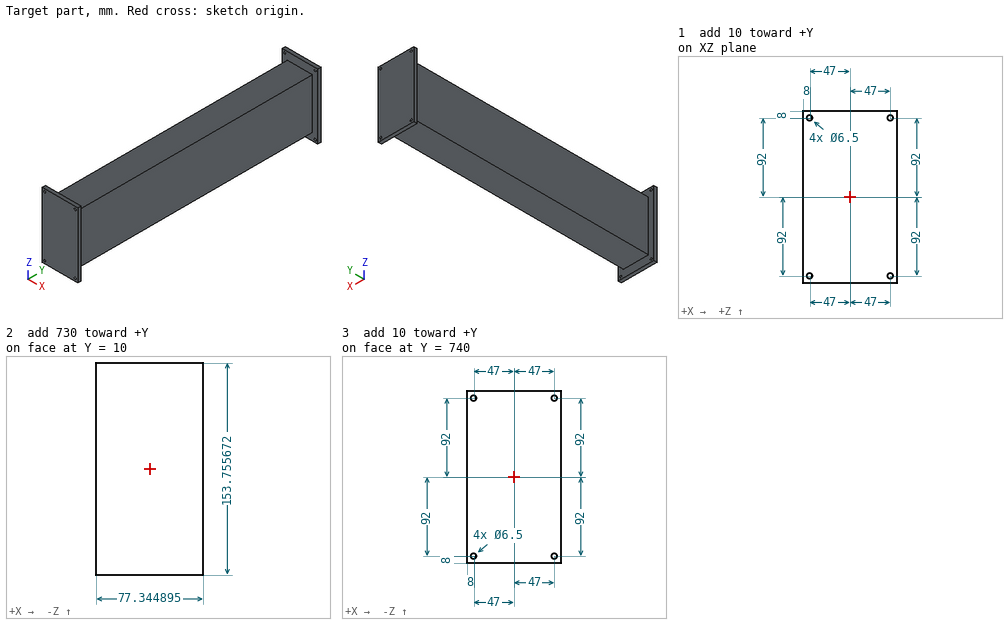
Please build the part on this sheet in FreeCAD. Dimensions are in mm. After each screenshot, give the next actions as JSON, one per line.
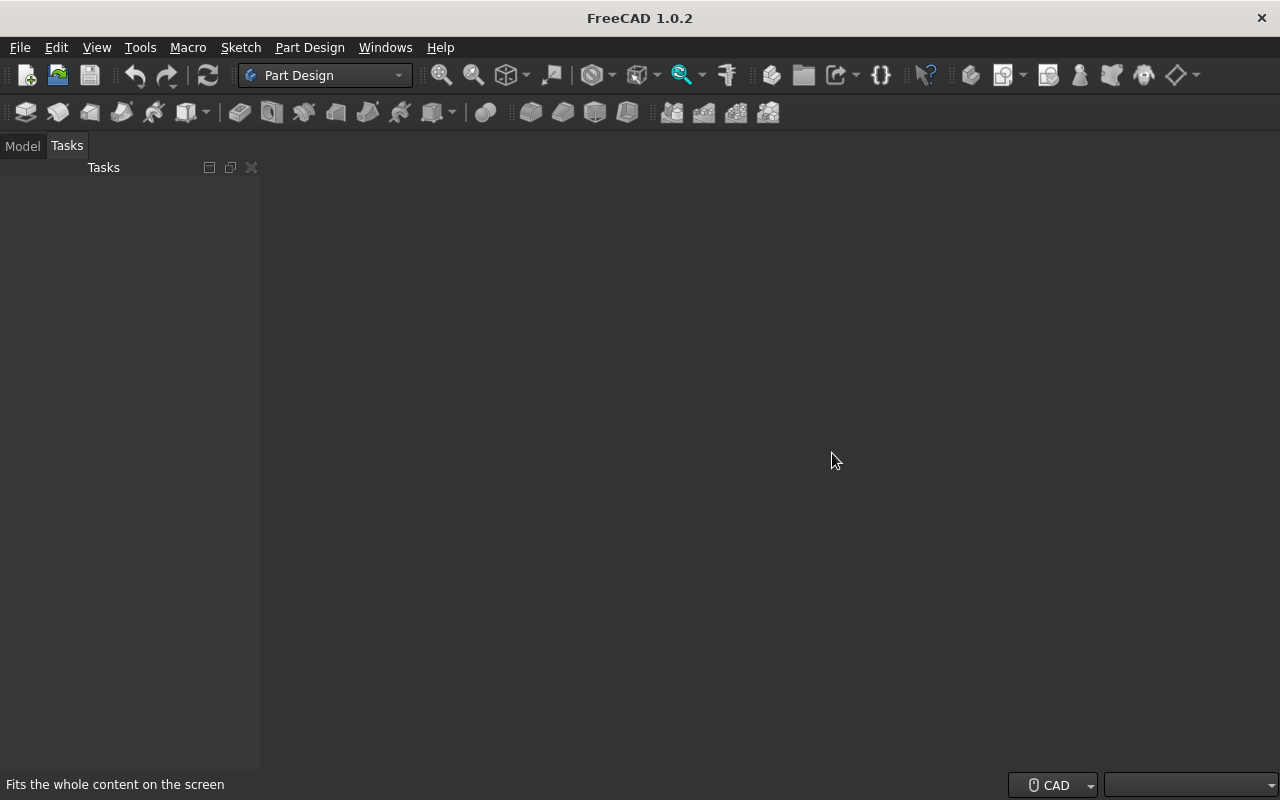
{"action": "left_click", "coordinate": [26, 76]}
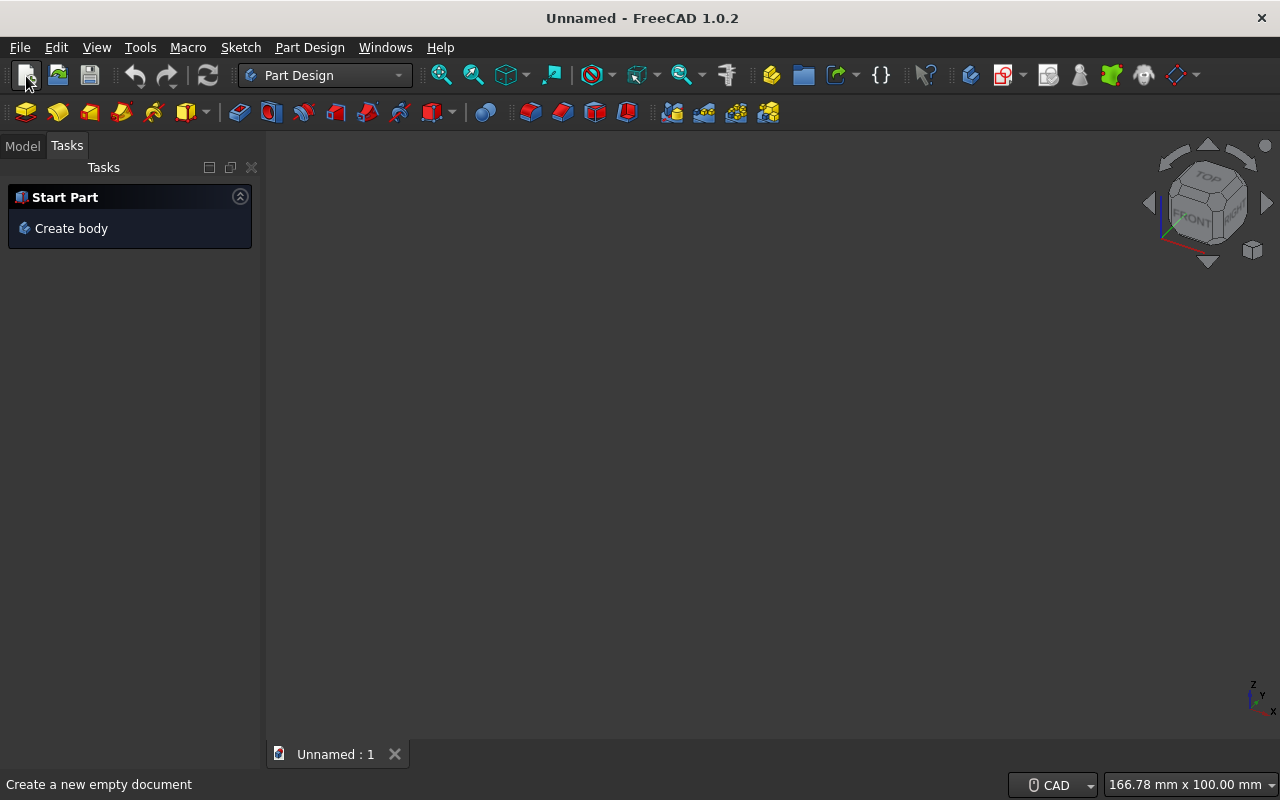
{"action": "left_click", "coordinate": [1004, 76]}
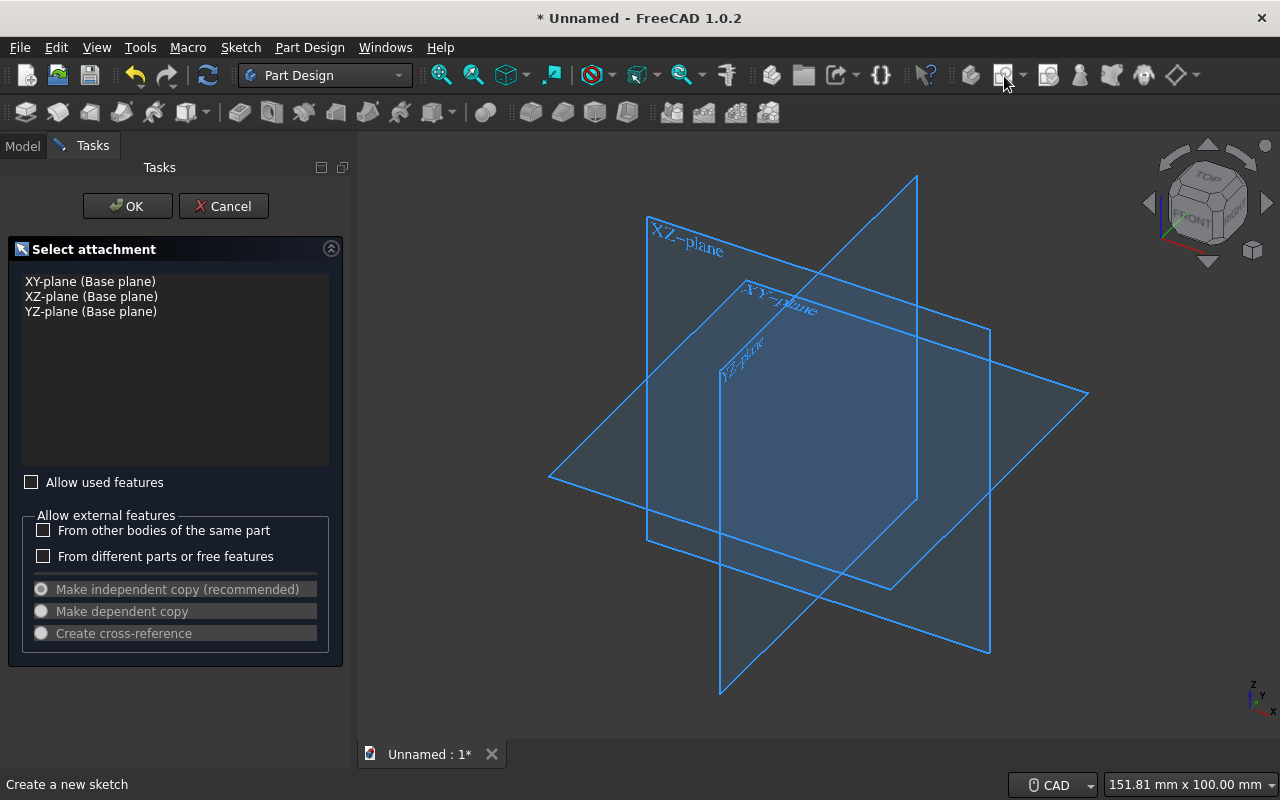
{"action": "left_click", "coordinate": [82, 296]}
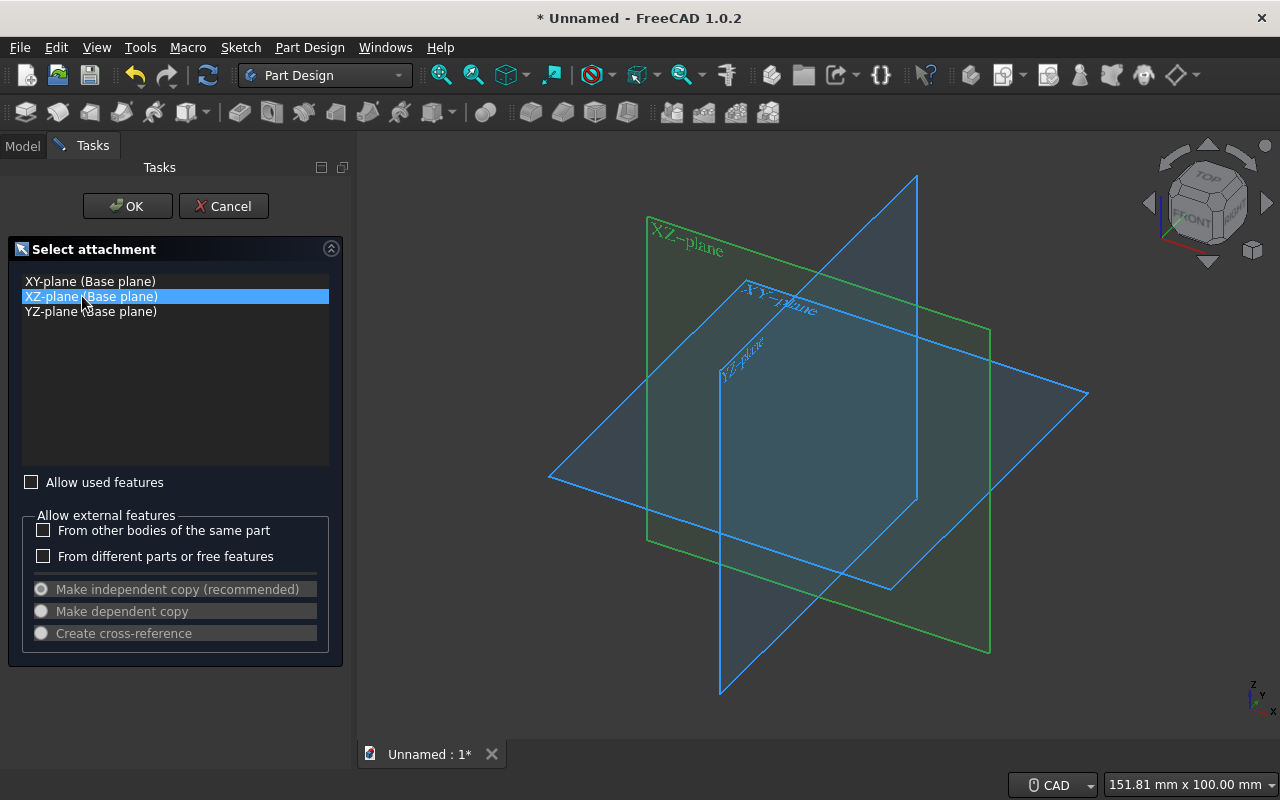
{"action": "left_click", "coordinate": [128, 206]}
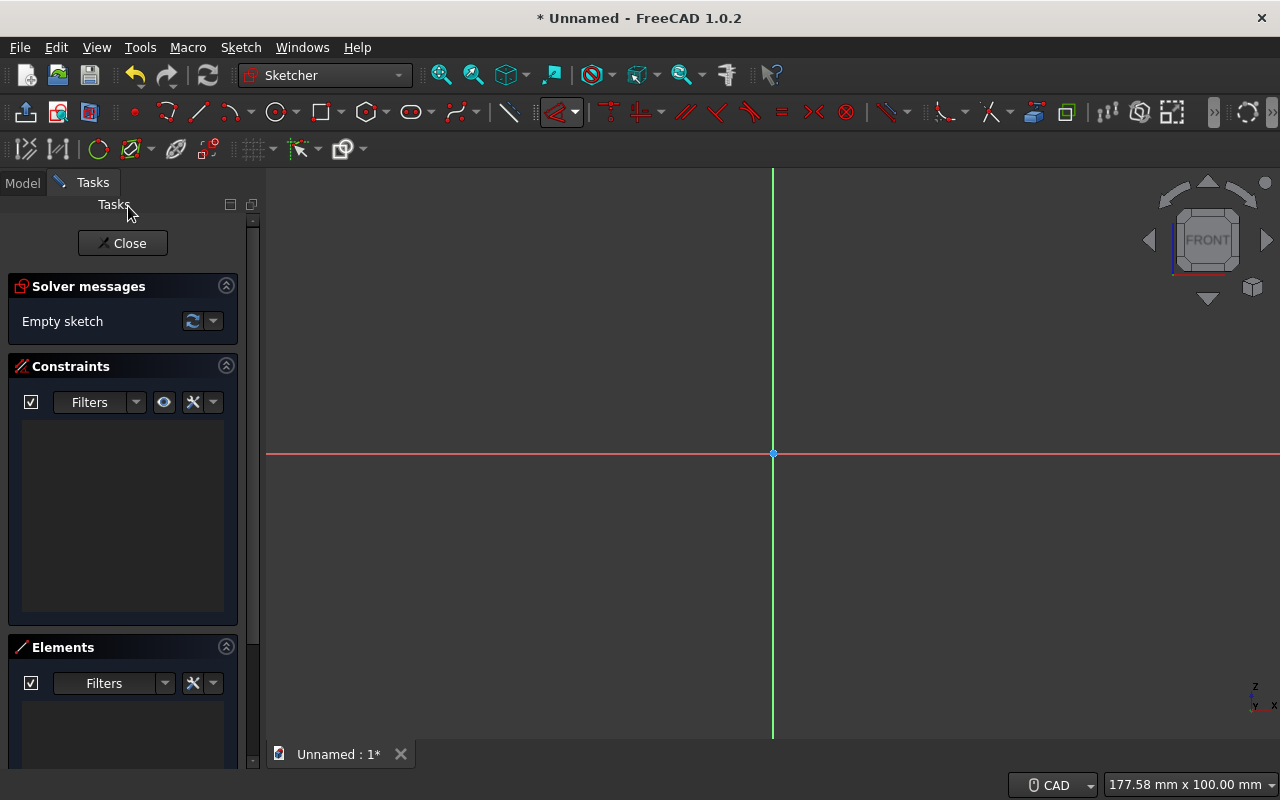
{"action": "scroll", "coordinate": [675, 453], "scroll_direction": "down", "scroll_amount": 6}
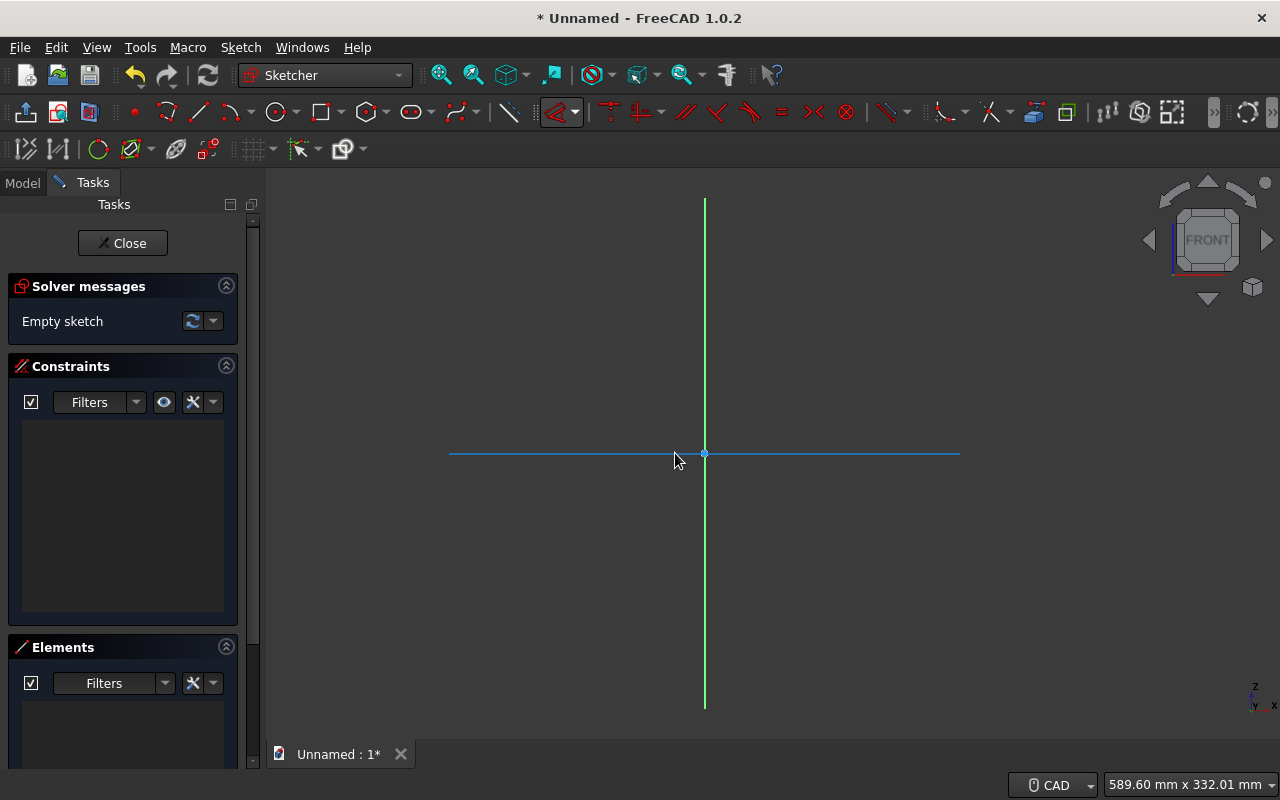
{"action": "left_click", "coordinate": [344, 112]}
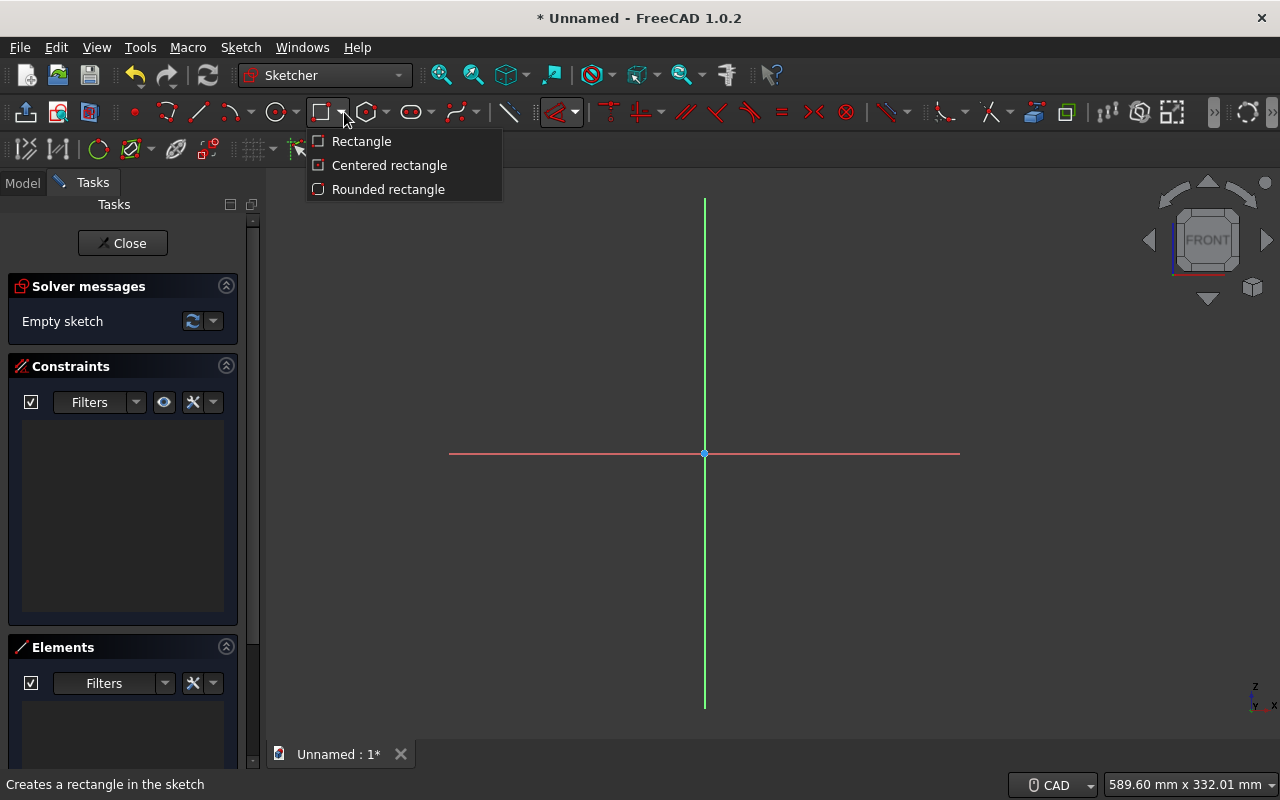
{"action": "left_click", "coordinate": [404, 165]}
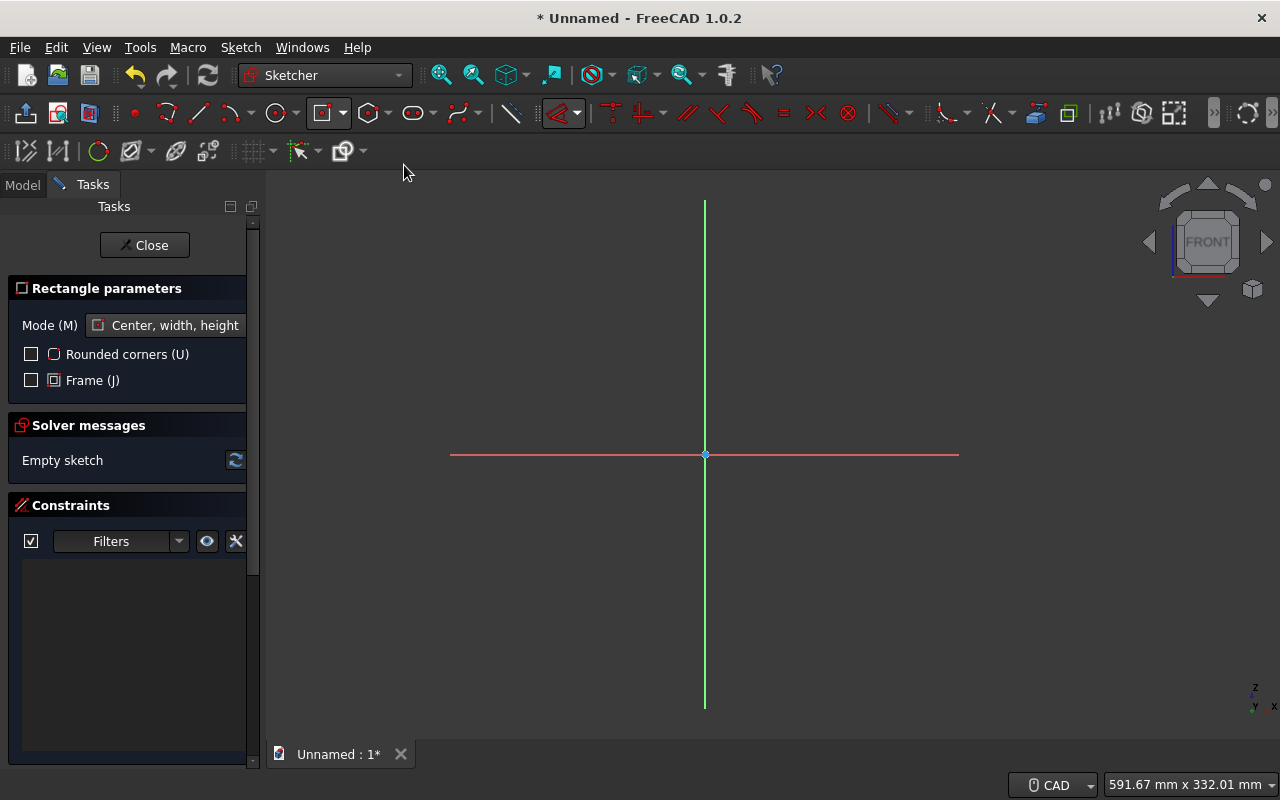
{"action": "left_click", "coordinate": [705, 454]}
{"action": "left_click", "coordinate": [799, 283]}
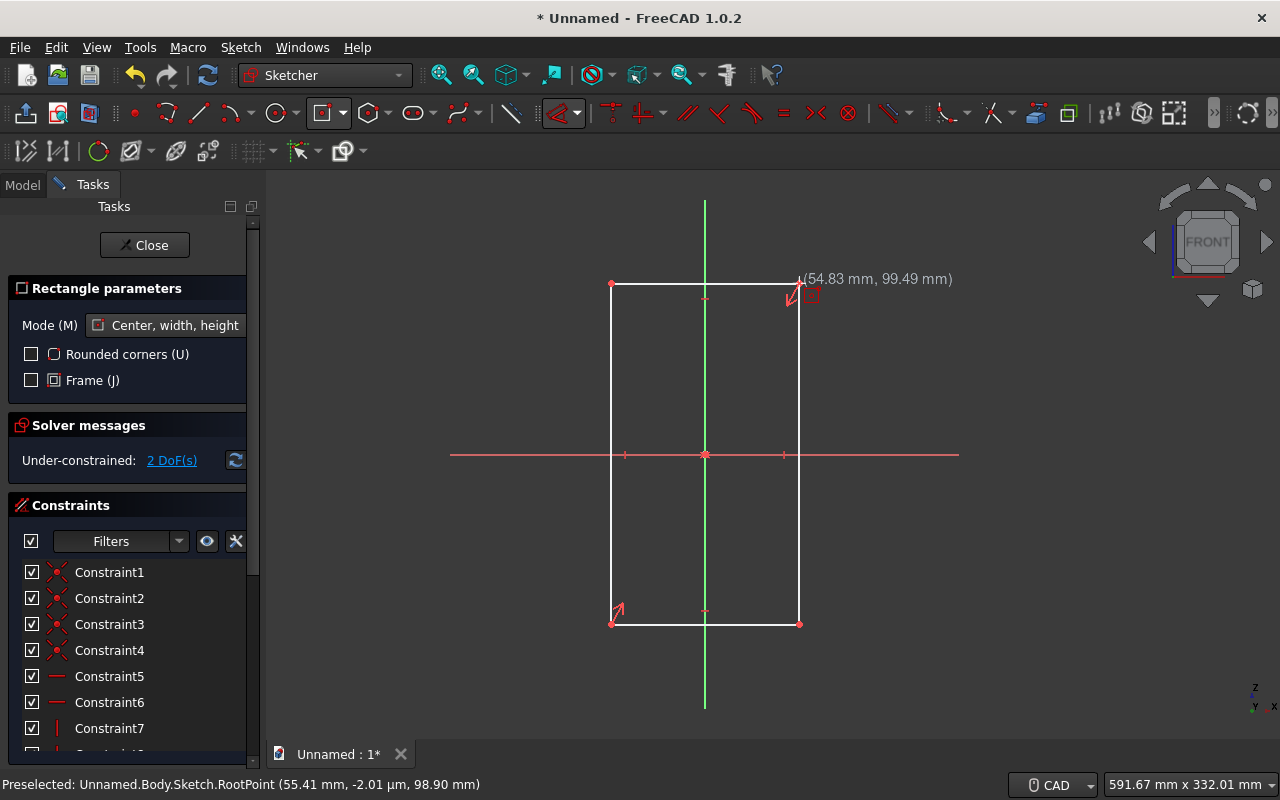
{"action": "left_click", "coordinate": [276, 114]}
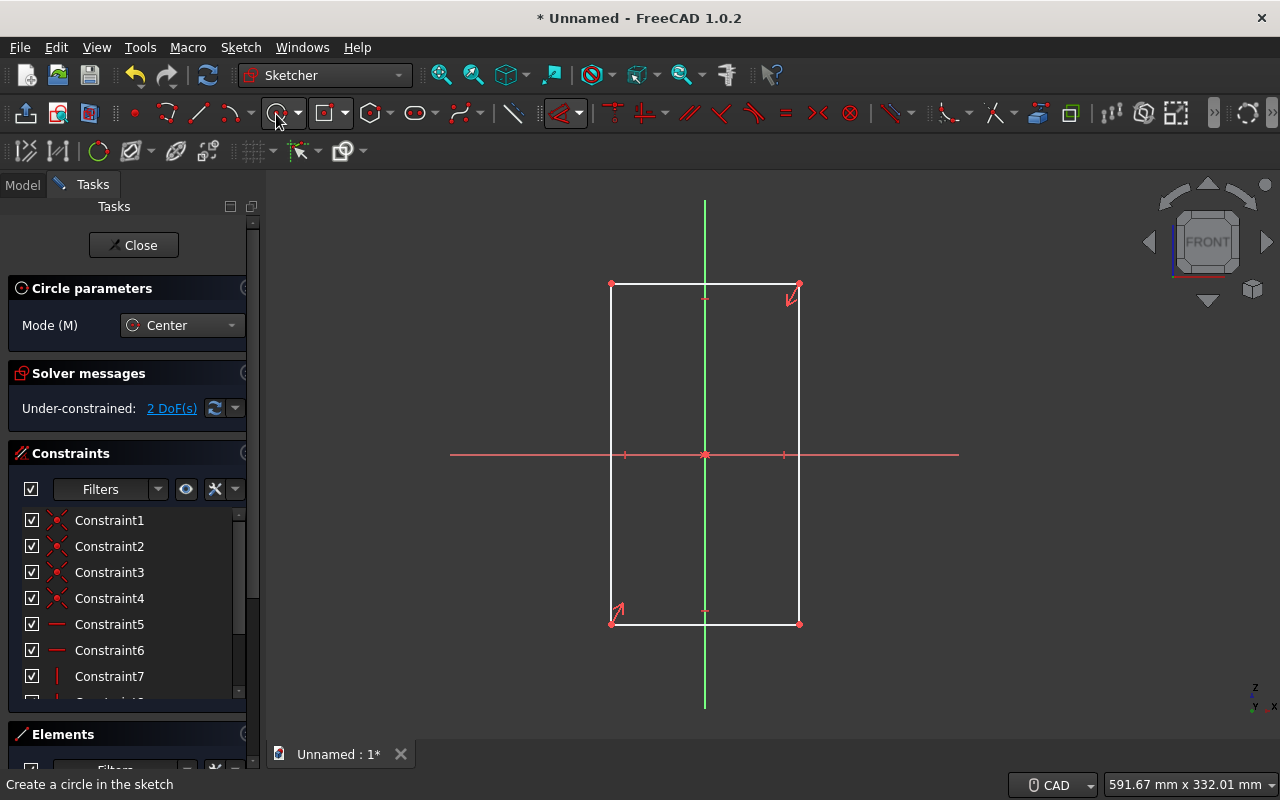
{"action": "scroll", "coordinate": [624, 297], "scroll_direction": "up", "scroll_amount": 8}